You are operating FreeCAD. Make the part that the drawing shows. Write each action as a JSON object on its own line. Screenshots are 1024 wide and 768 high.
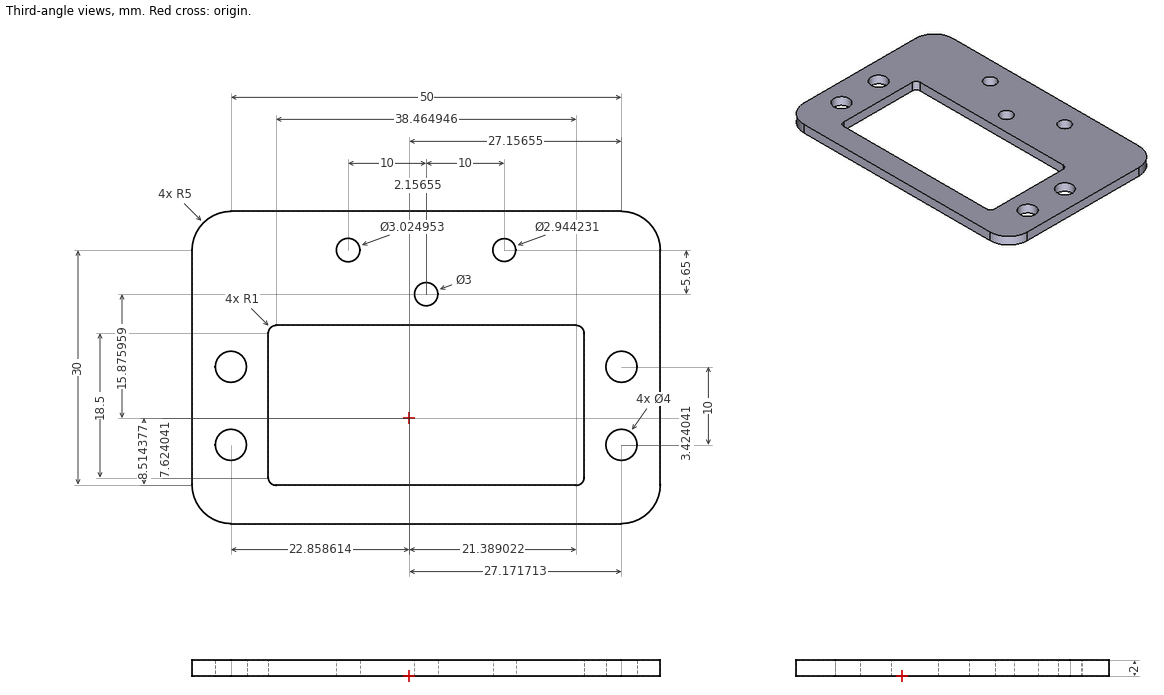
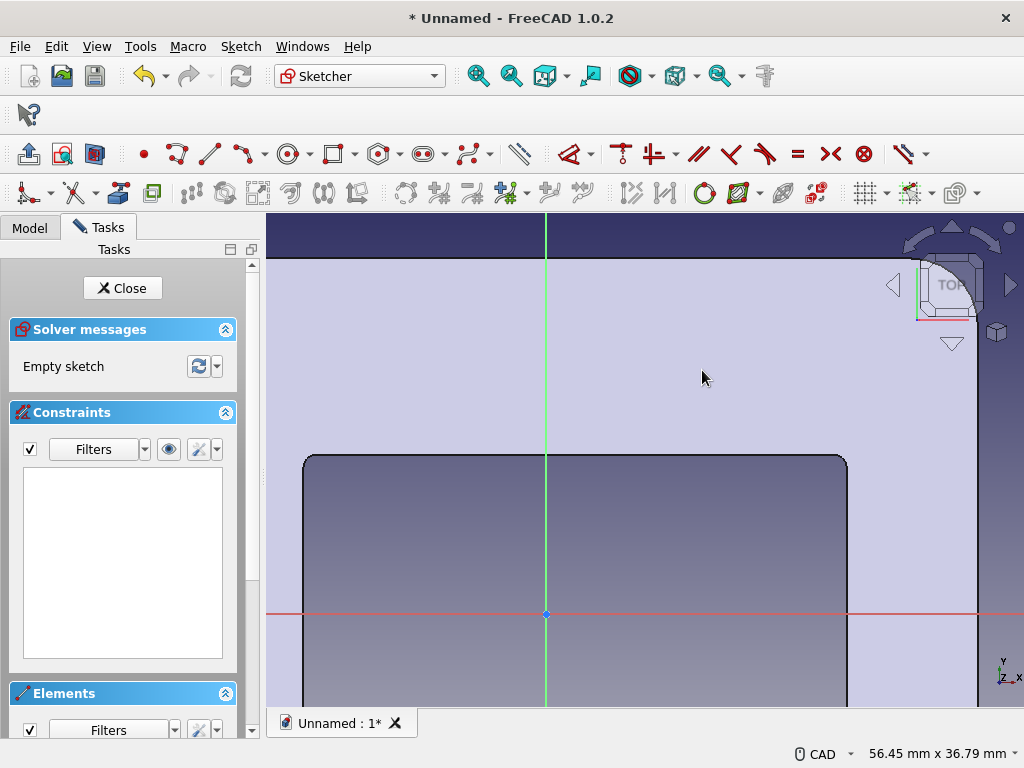
{"action": "left_click", "coordinate": [288, 154]}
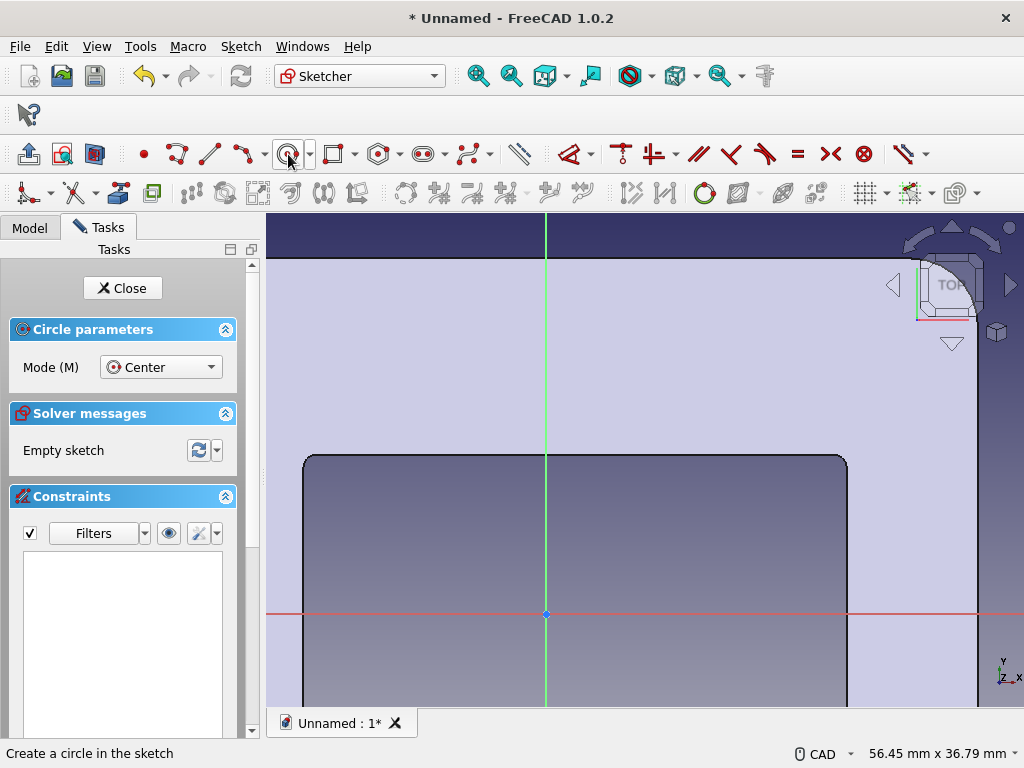
{"action": "left_click", "coordinate": [575, 401]}
{"action": "left_click", "coordinate": [589, 387]}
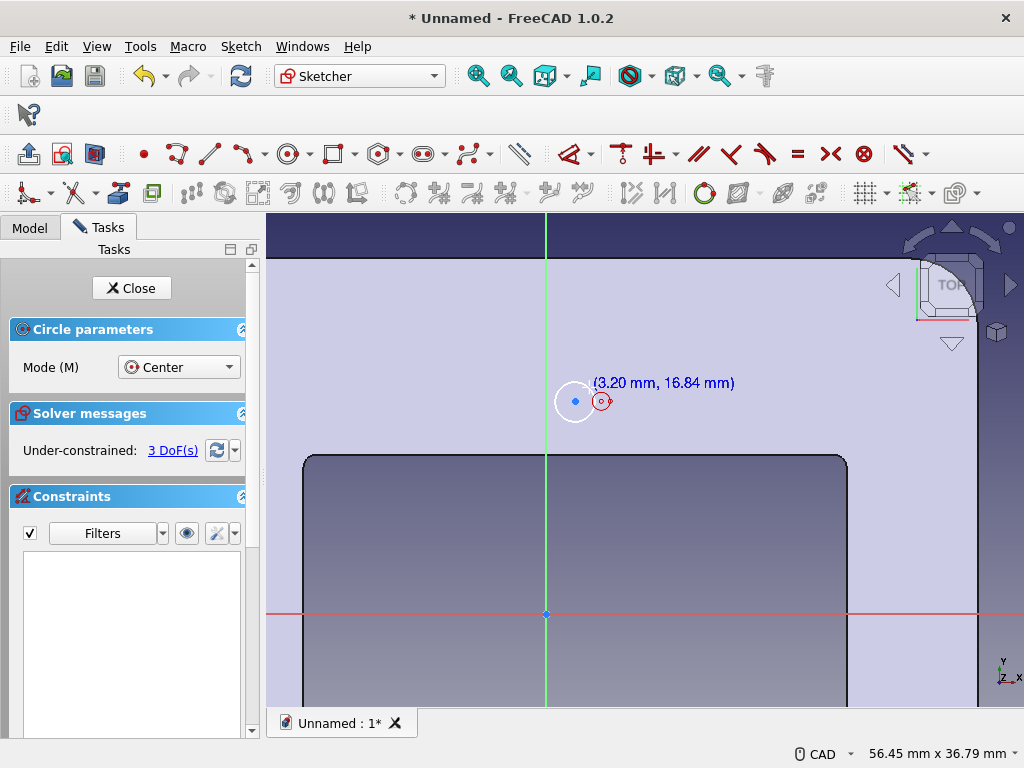
{"action": "left_click", "coordinate": [709, 325]}
{"action": "left_click", "coordinate": [723, 311]}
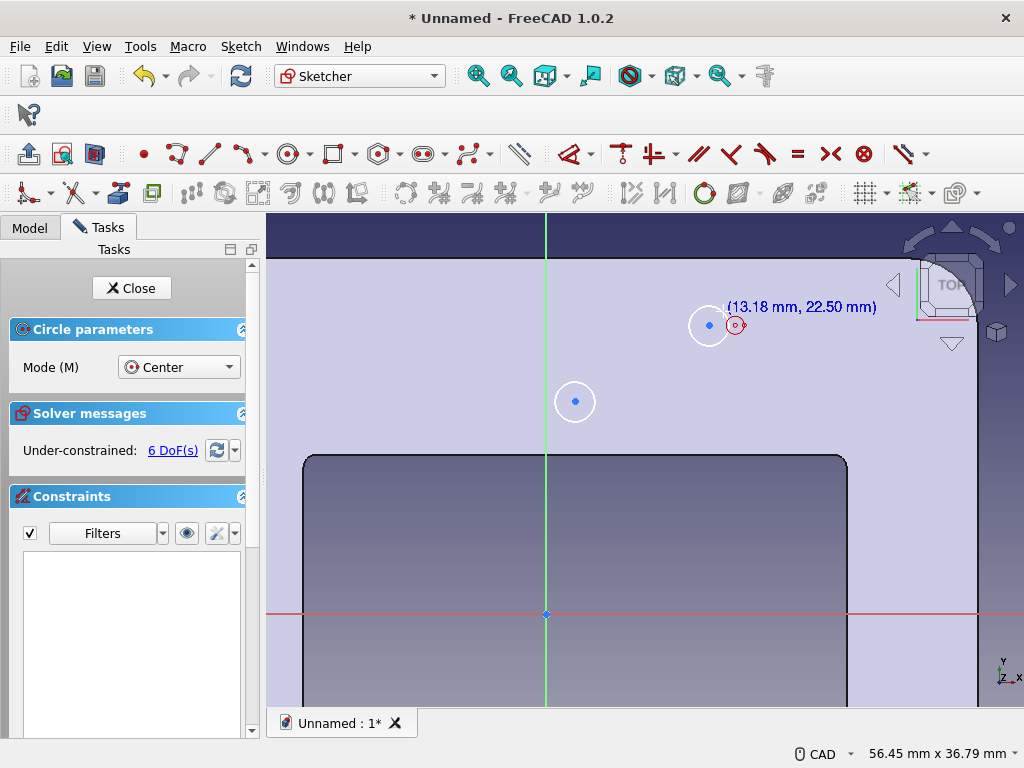
{"action": "left_click", "coordinate": [441, 325]}
{"action": "left_click", "coordinate": [455, 311]}
{"action": "key", "text": "Escape"}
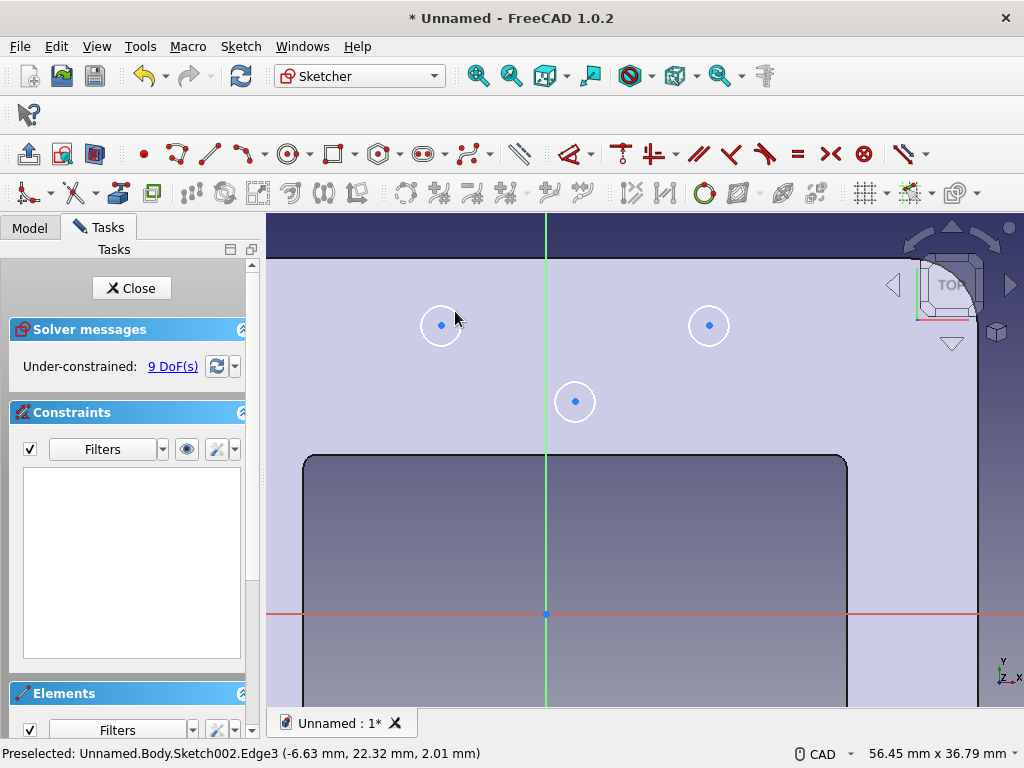
{"action": "left_click", "coordinate": [568, 154]}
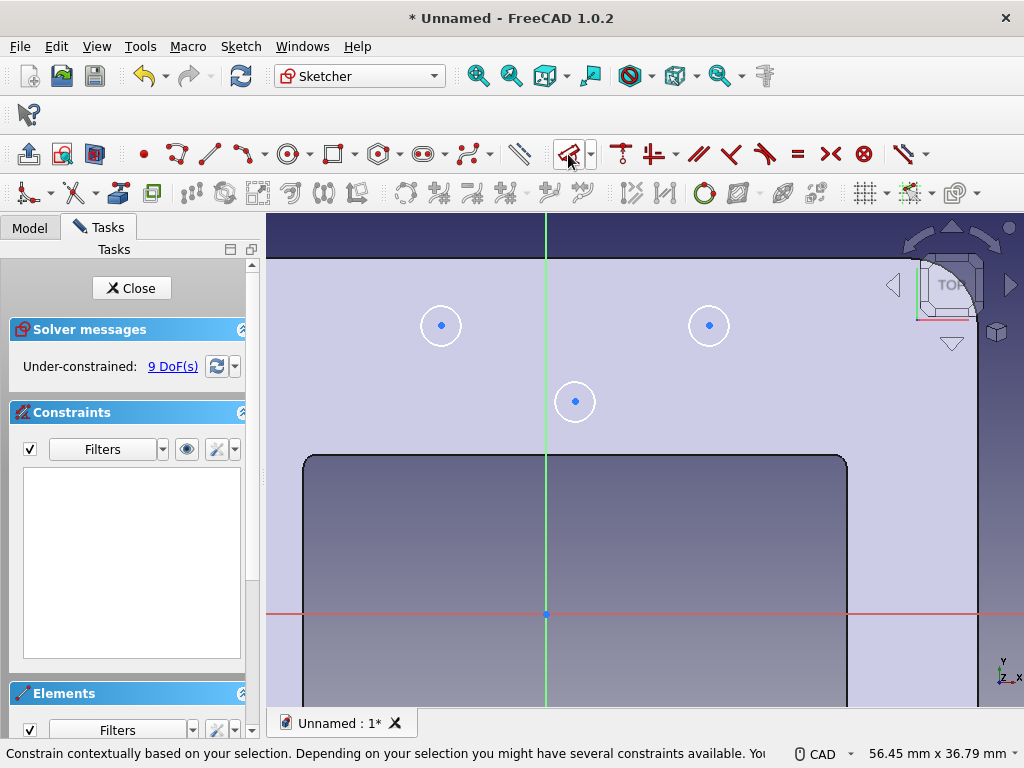
{"action": "left_click", "coordinate": [589, 388]}
{"action": "left_click", "coordinate": [612, 365]}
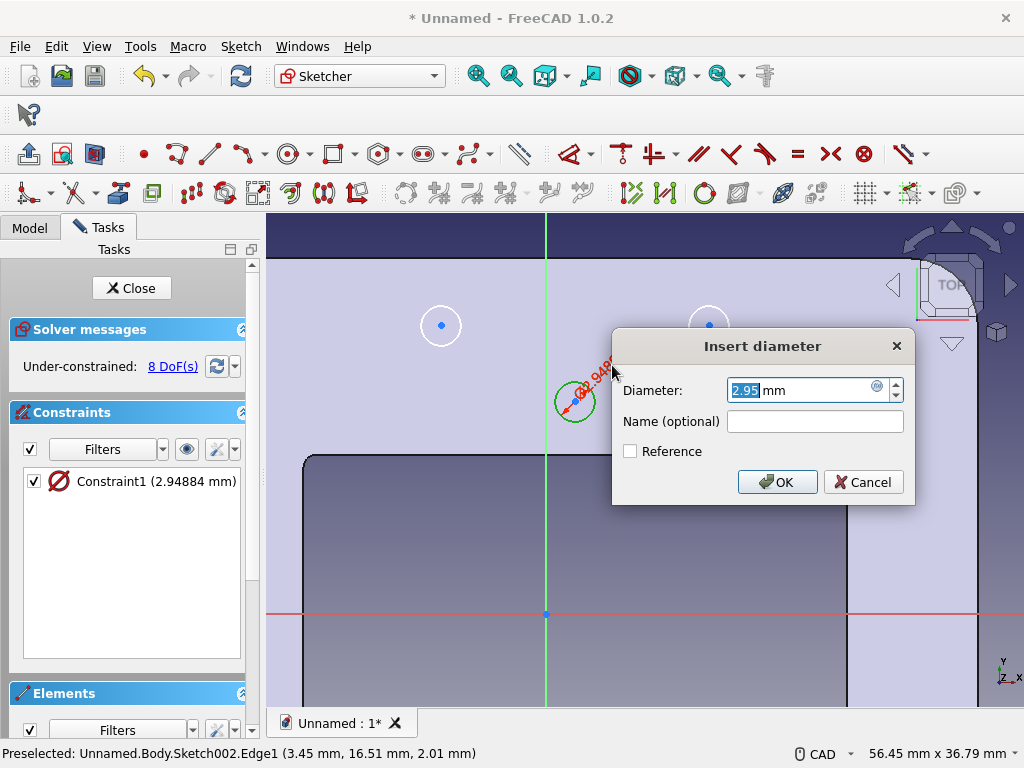
{"action": "type", "text": "3"}
{"action": "key", "text": "Return"}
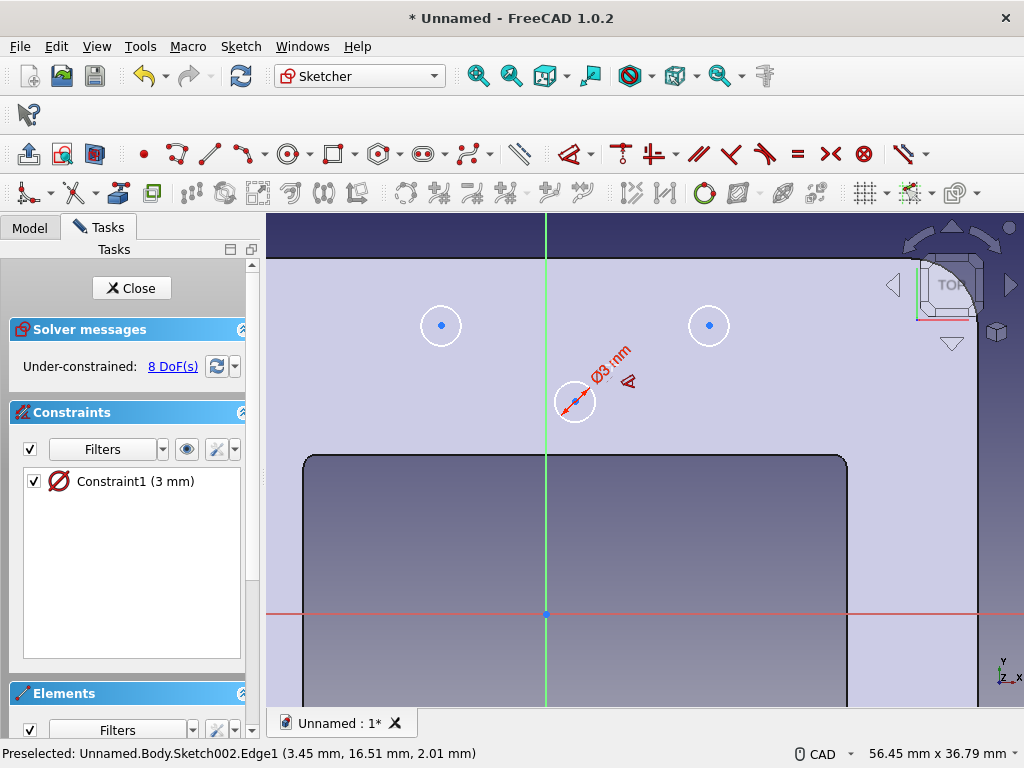
{"action": "left_click", "coordinate": [723, 312]}
{"action": "left_click", "coordinate": [746, 289]}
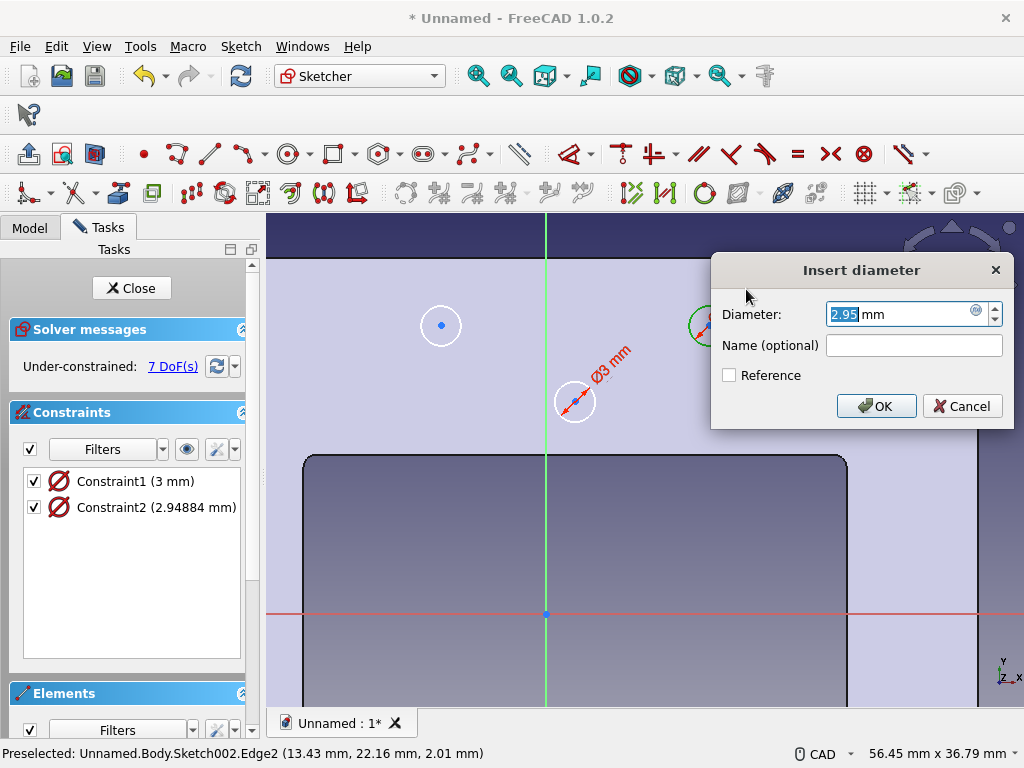
{"action": "type", "text": "2.944231"}
{"action": "key", "text": "Return"}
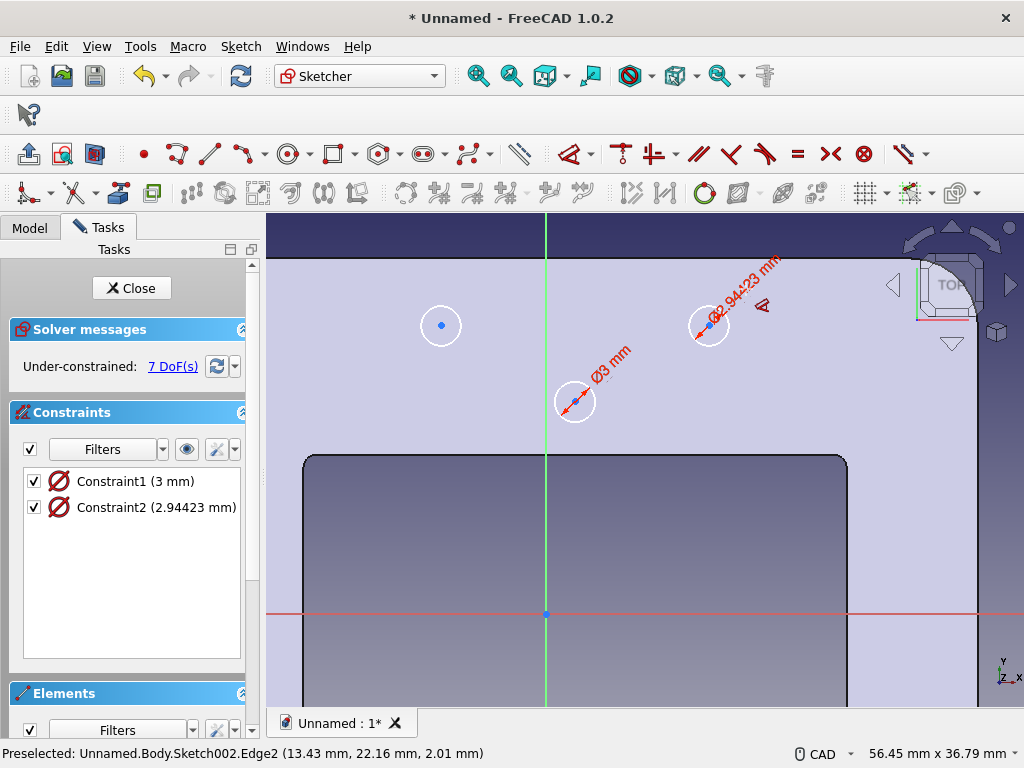
{"action": "left_click", "coordinate": [455, 312]}
{"action": "left_click", "coordinate": [478, 289]}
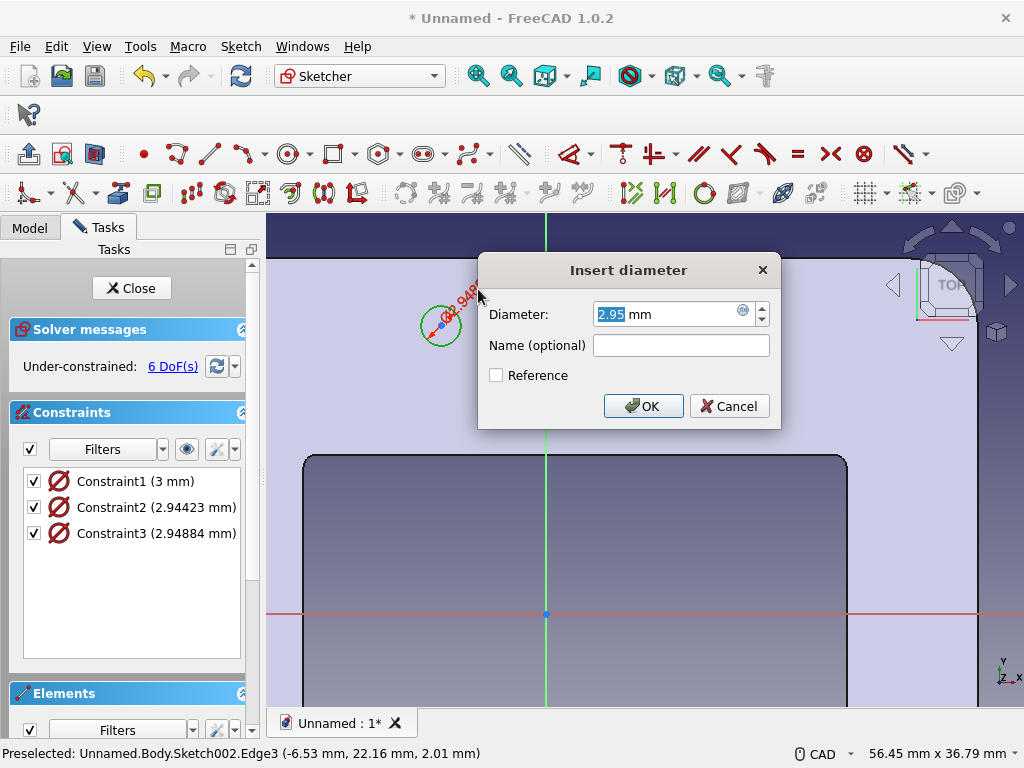
{"action": "type", "text": "3.024953"}
{"action": "key", "text": "Return"}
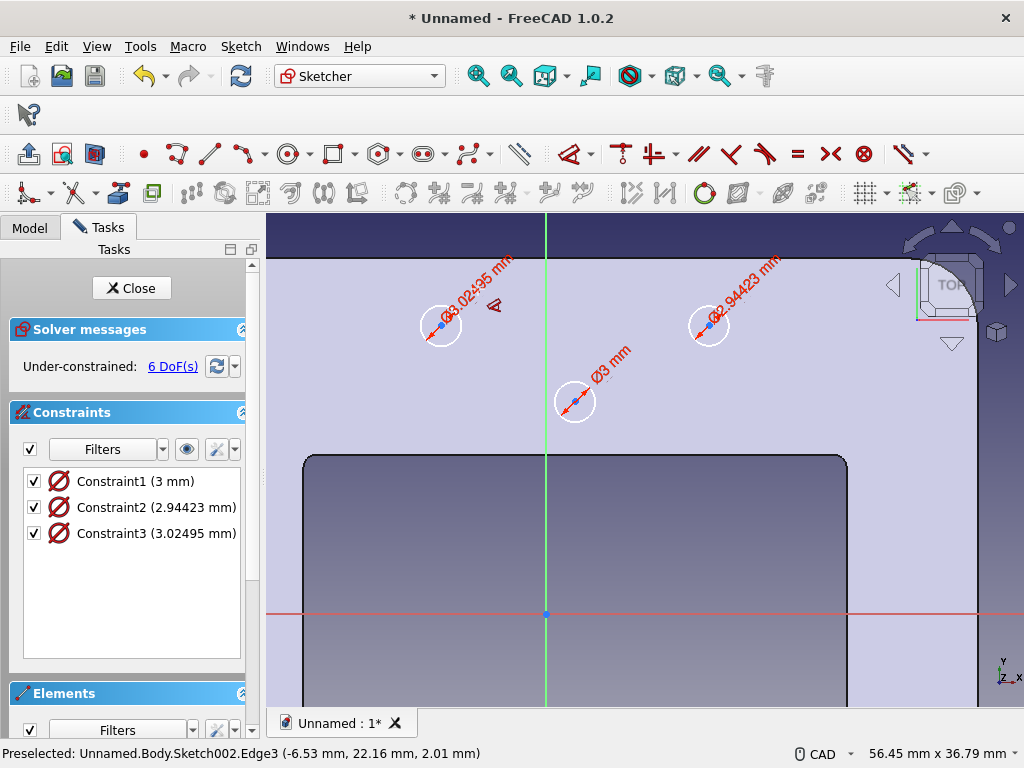
{"action": "left_click", "coordinate": [575, 402]}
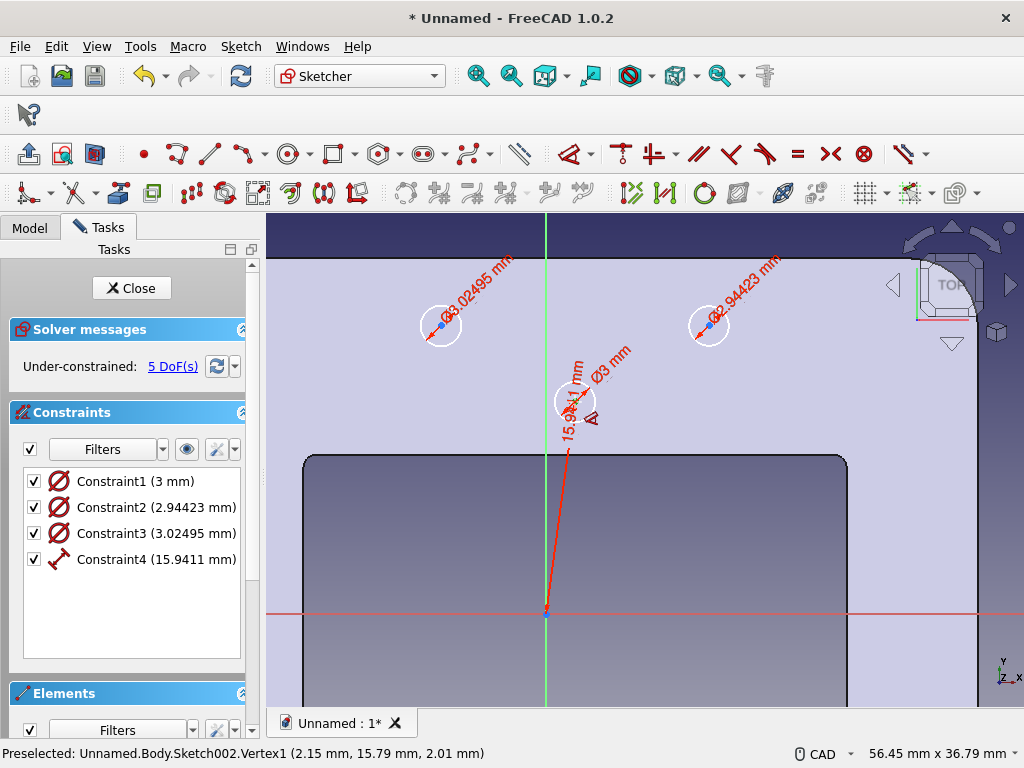
{"action": "left_click", "coordinate": [709, 326]}
{"action": "left_click", "coordinate": [642, 292]}